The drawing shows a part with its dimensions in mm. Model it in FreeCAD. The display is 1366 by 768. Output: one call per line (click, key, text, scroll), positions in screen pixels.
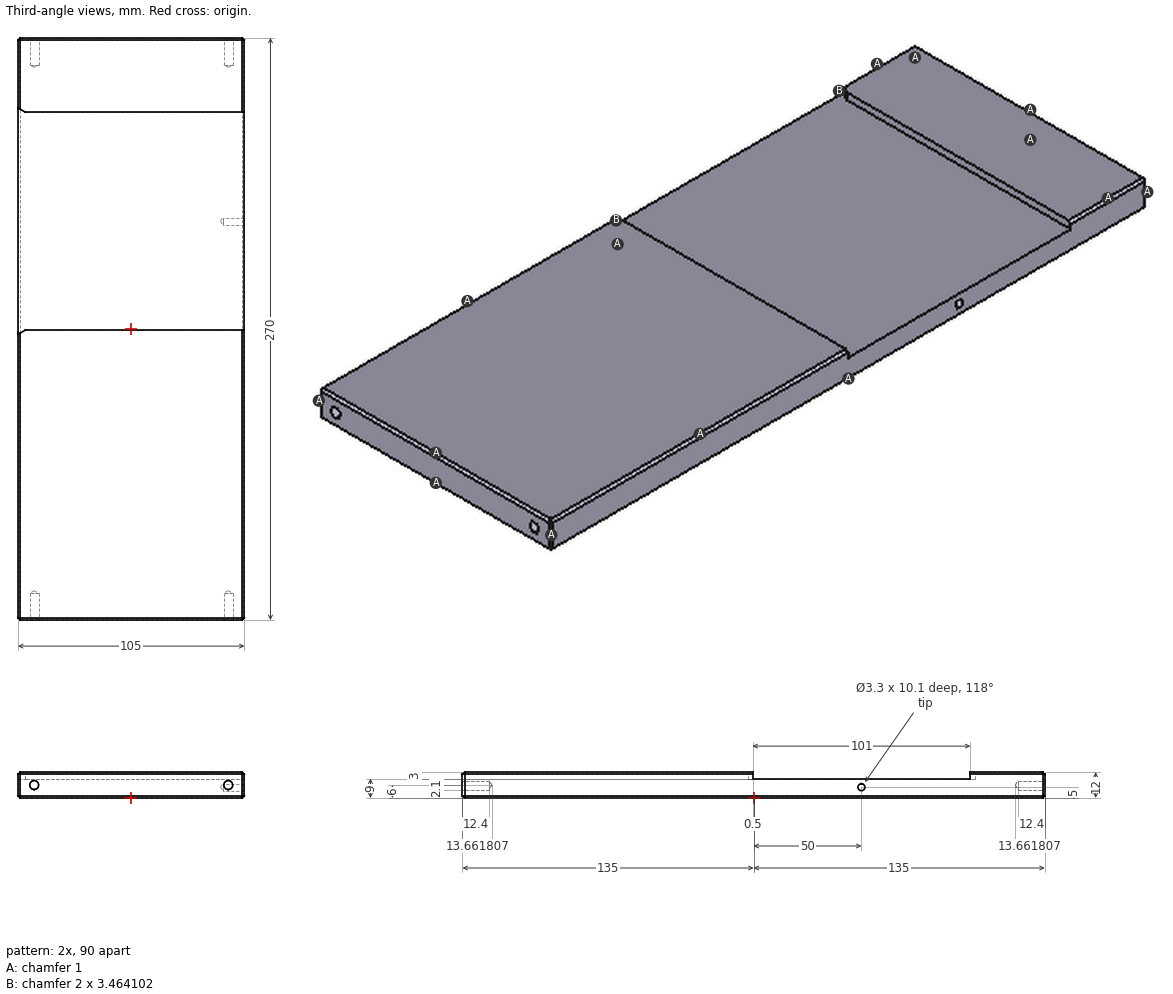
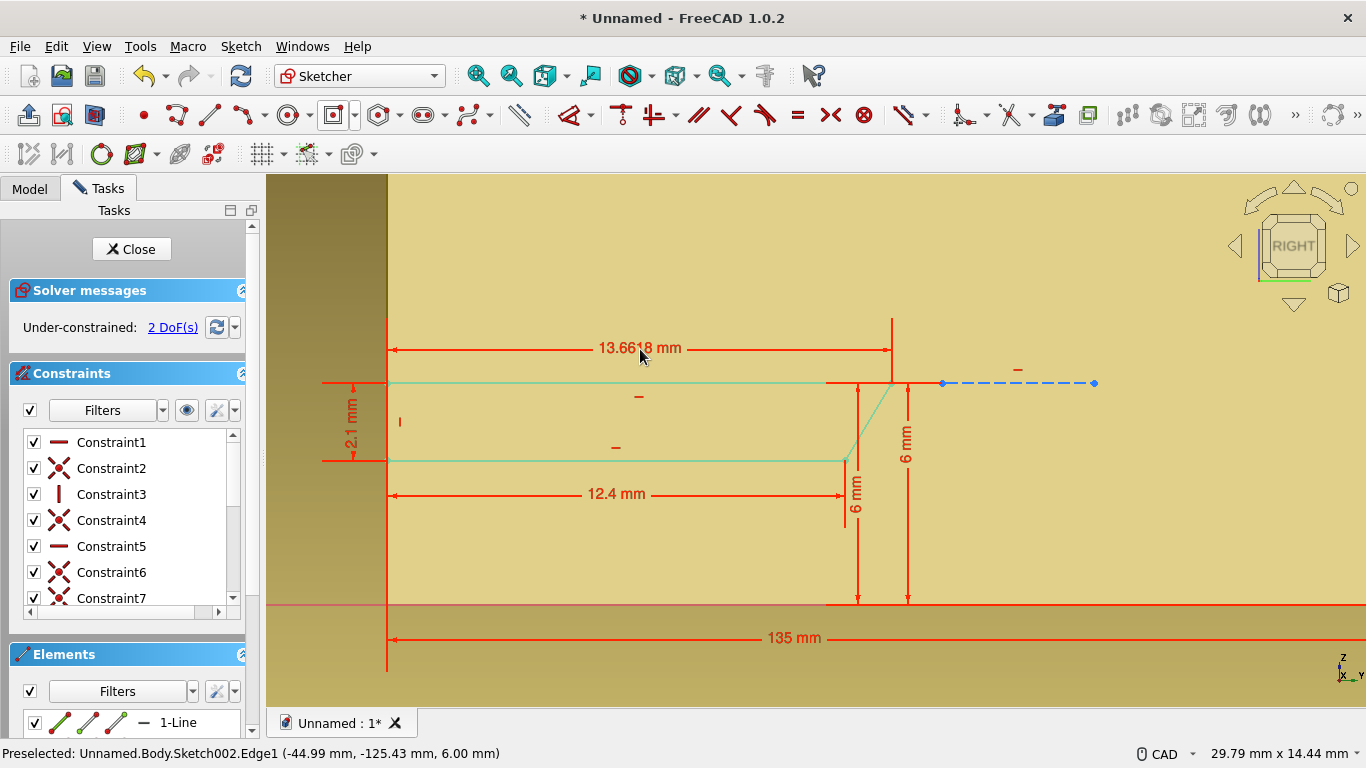
click(132, 249)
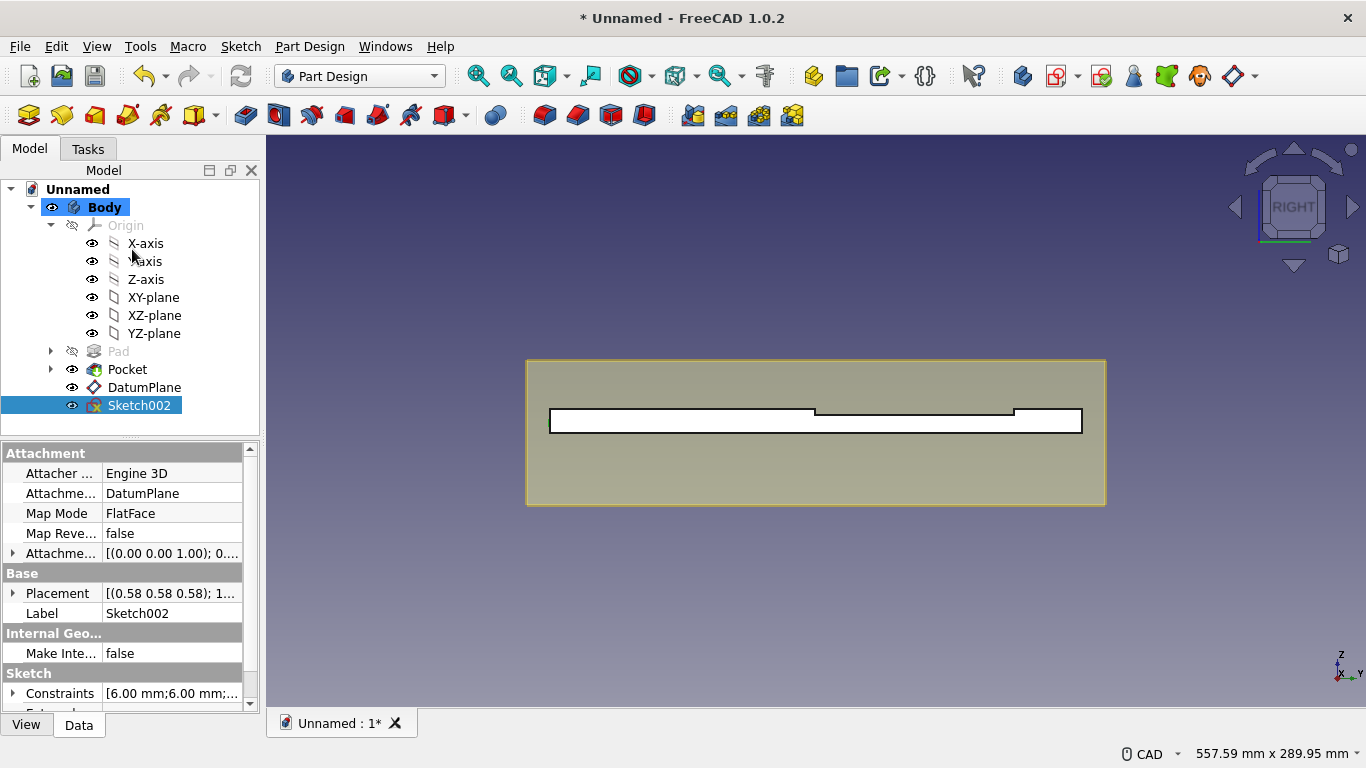
click(312, 116)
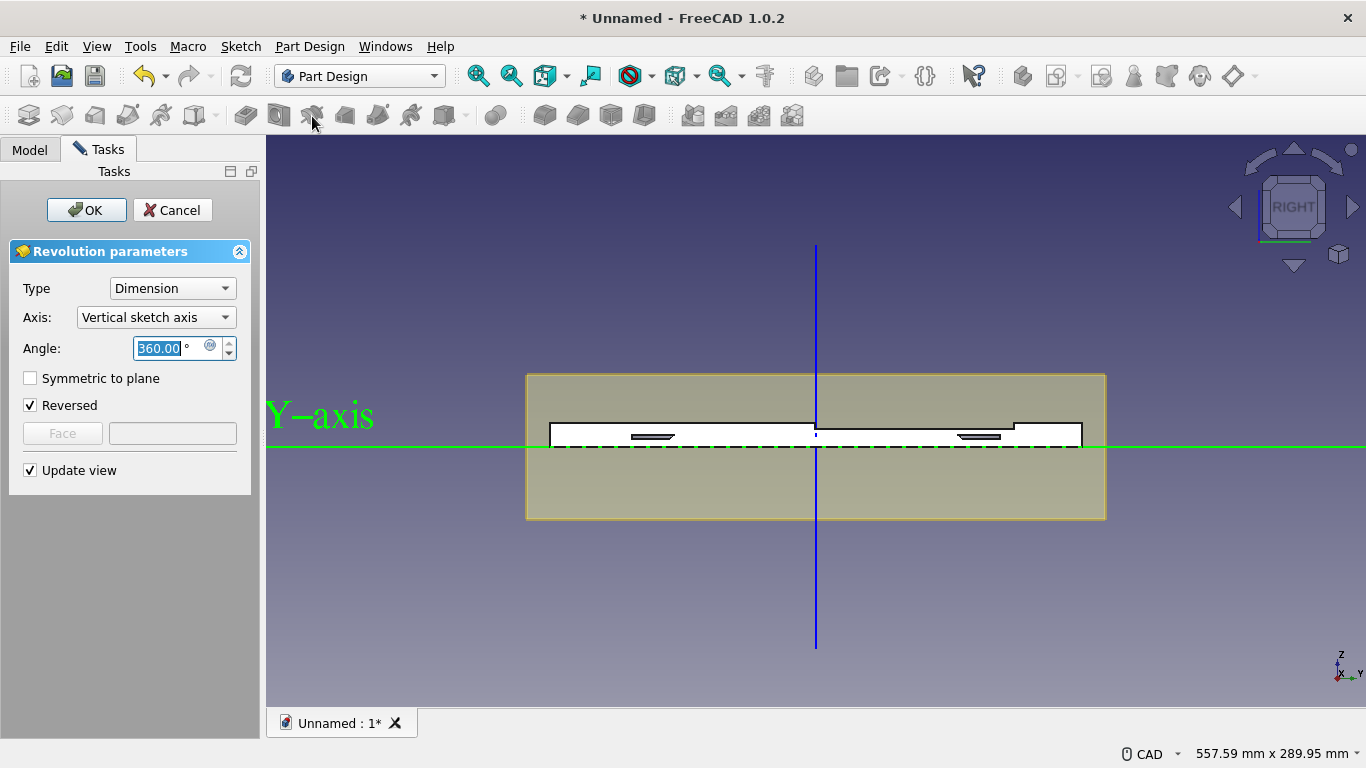
click(157, 318)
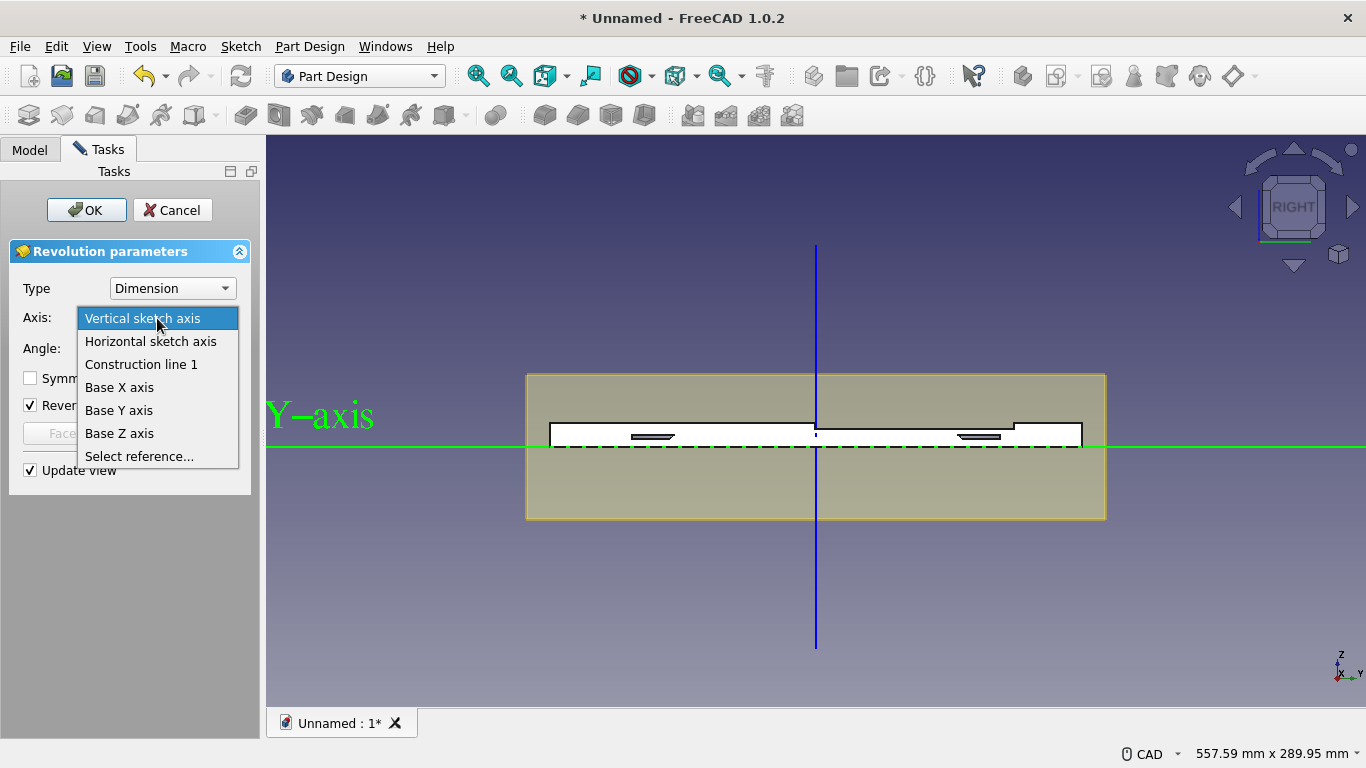
click(156, 364)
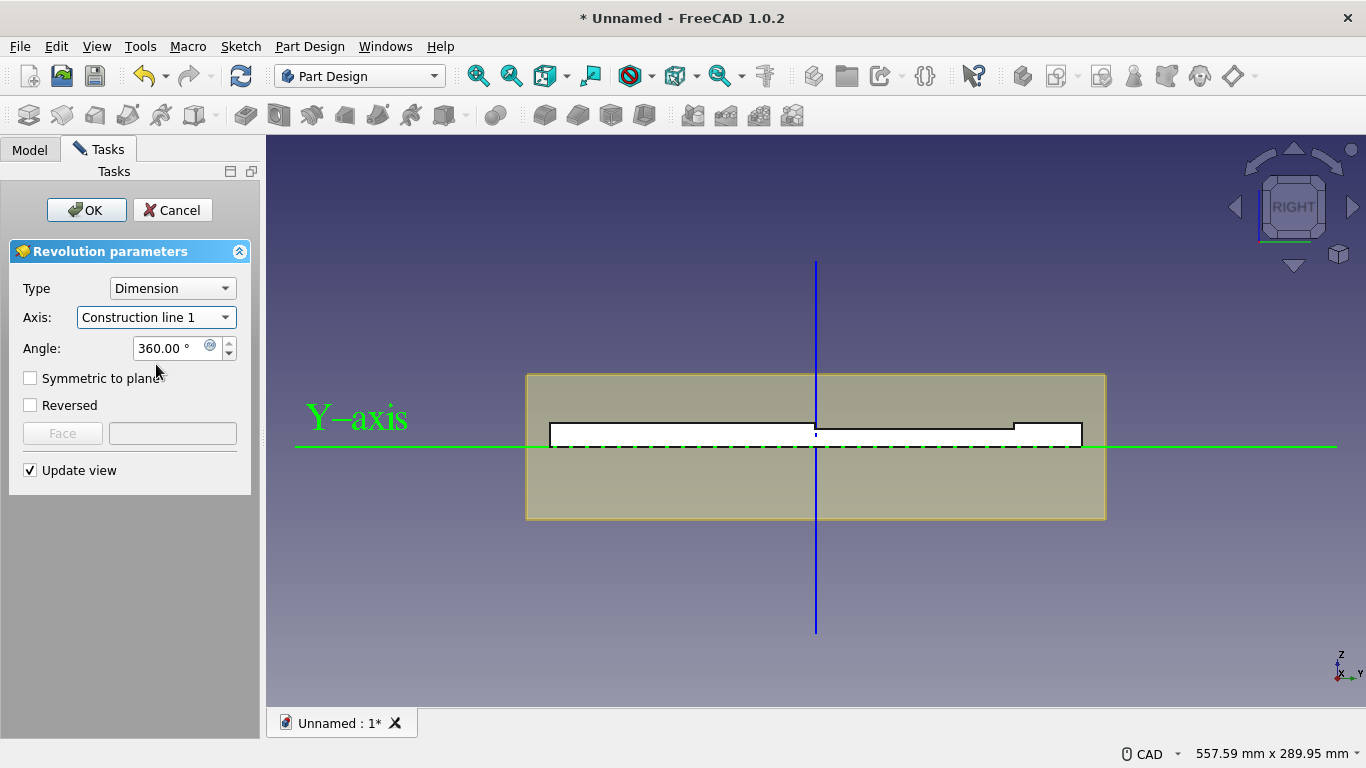
click(87, 210)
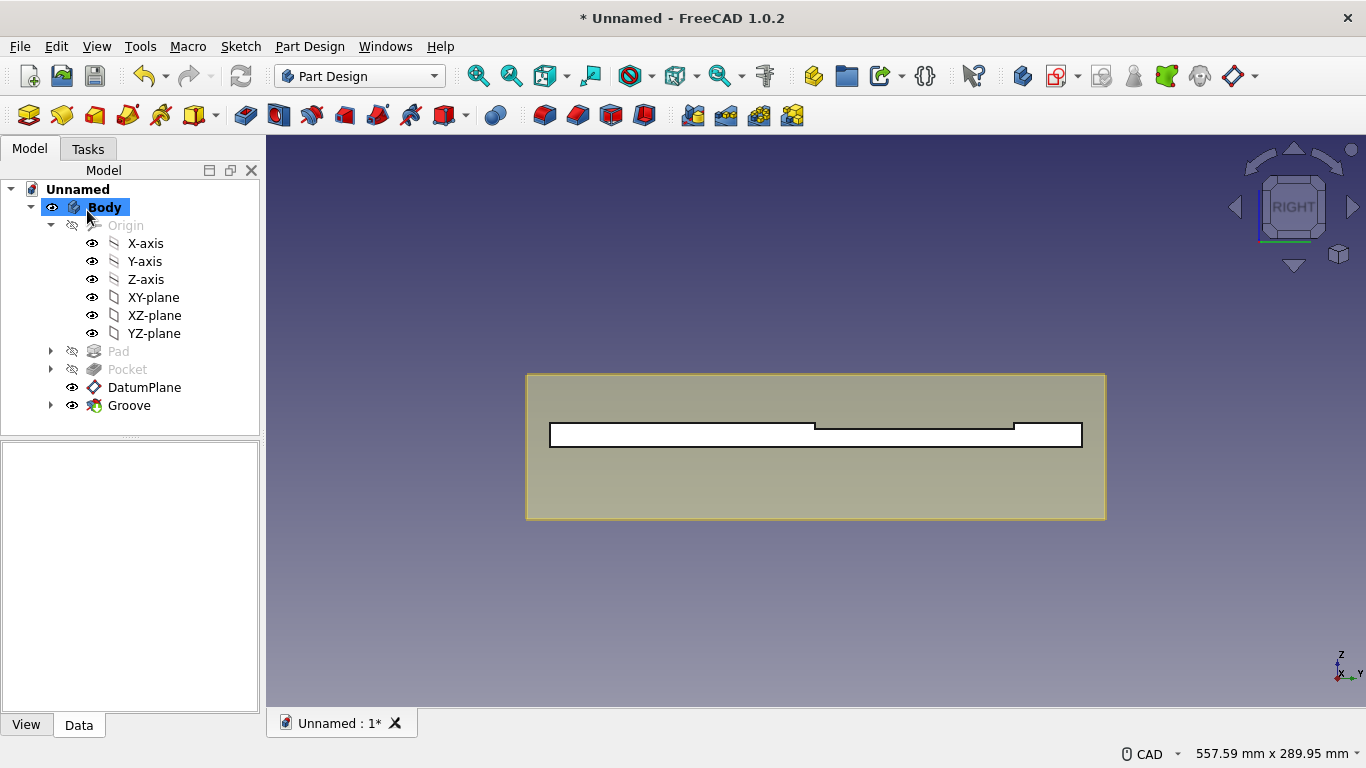
click(117, 387)
key(space)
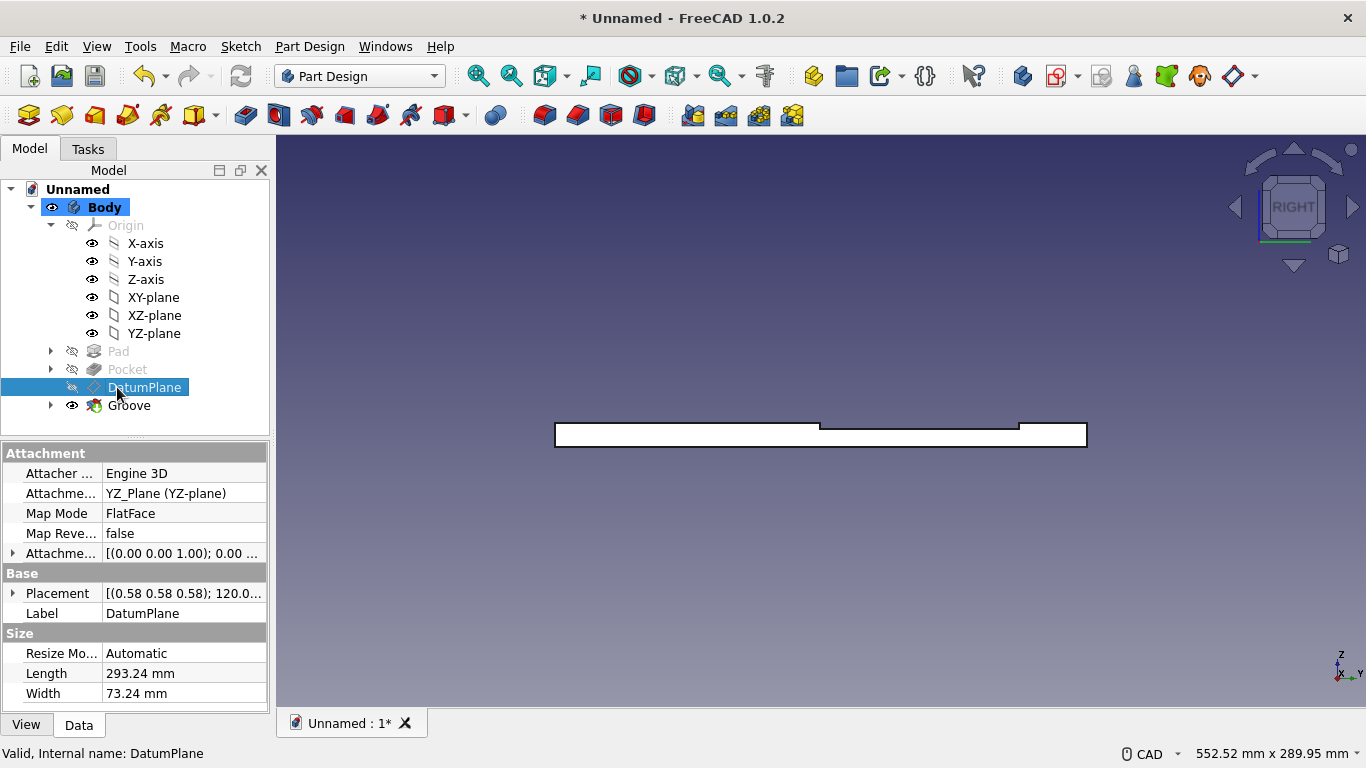
click(117, 405)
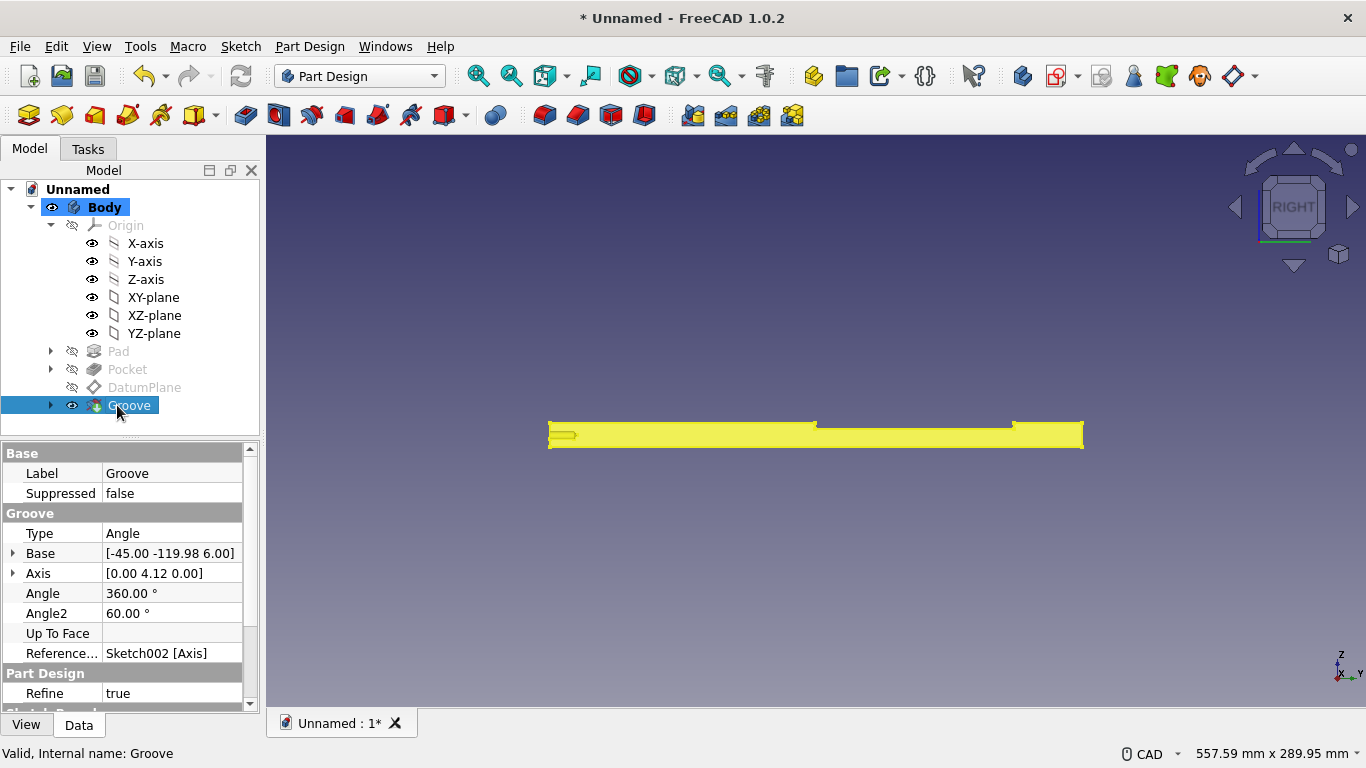
click(726, 116)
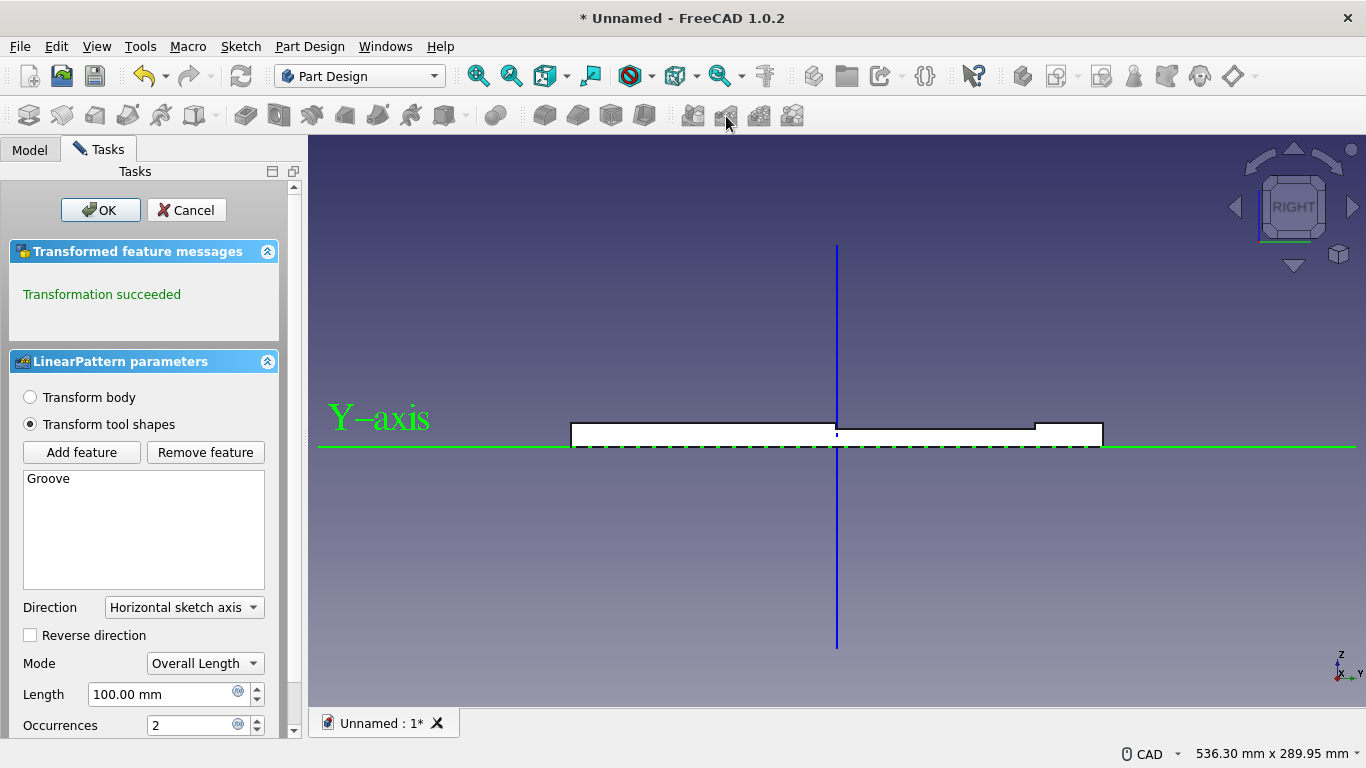
click(185, 608)